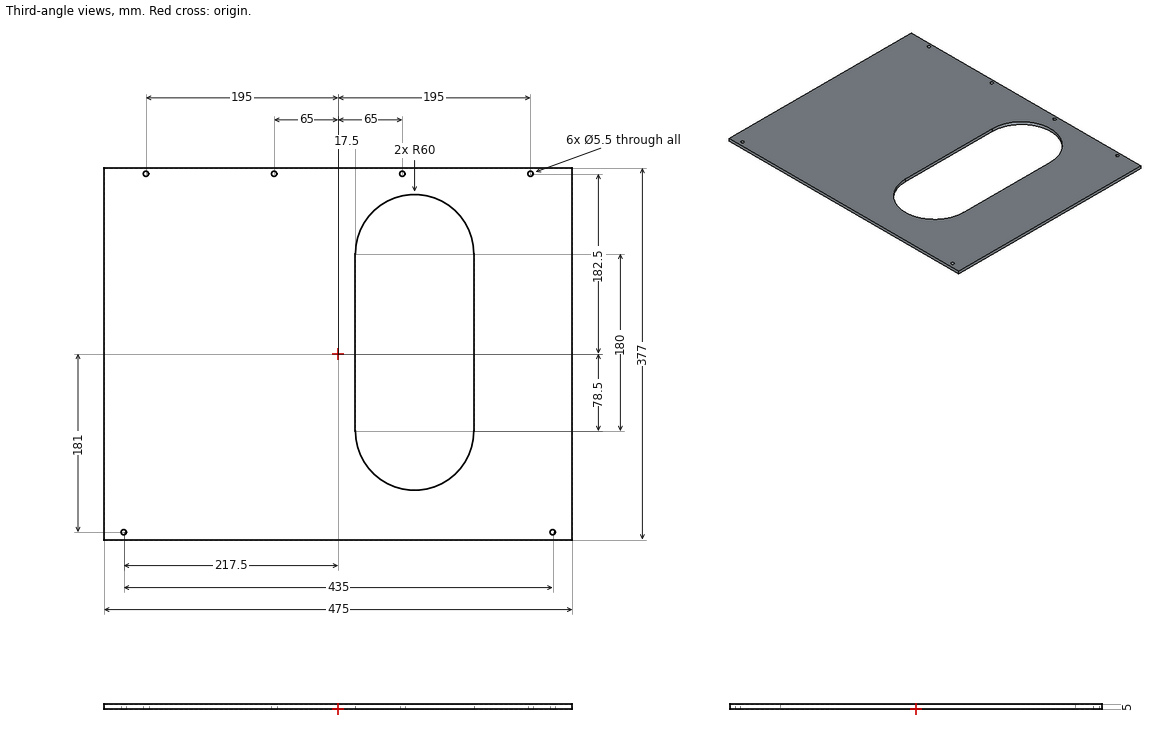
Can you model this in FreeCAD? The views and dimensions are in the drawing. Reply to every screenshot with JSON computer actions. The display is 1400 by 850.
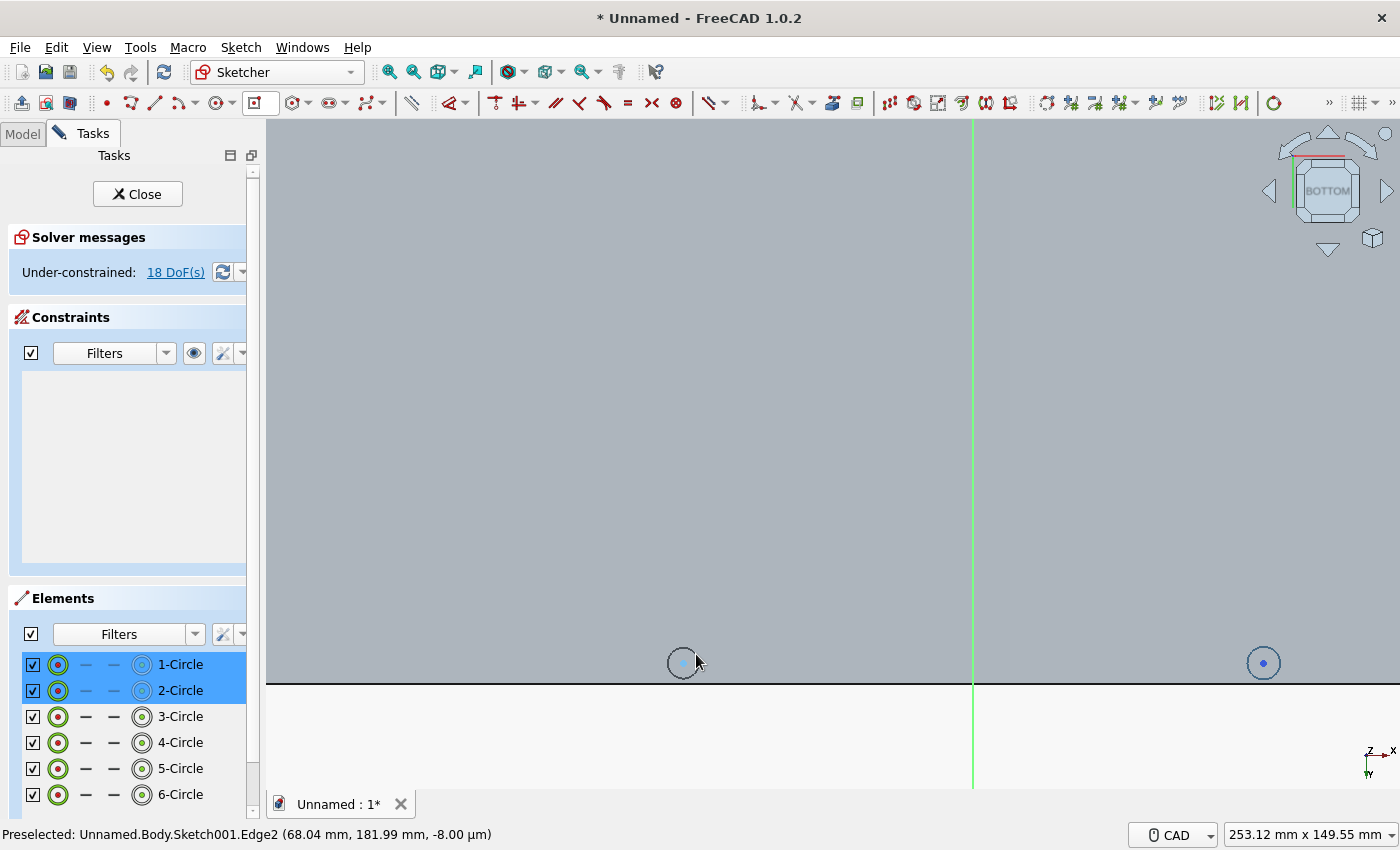
{"action": "left_click", "coordinate": [694, 652]}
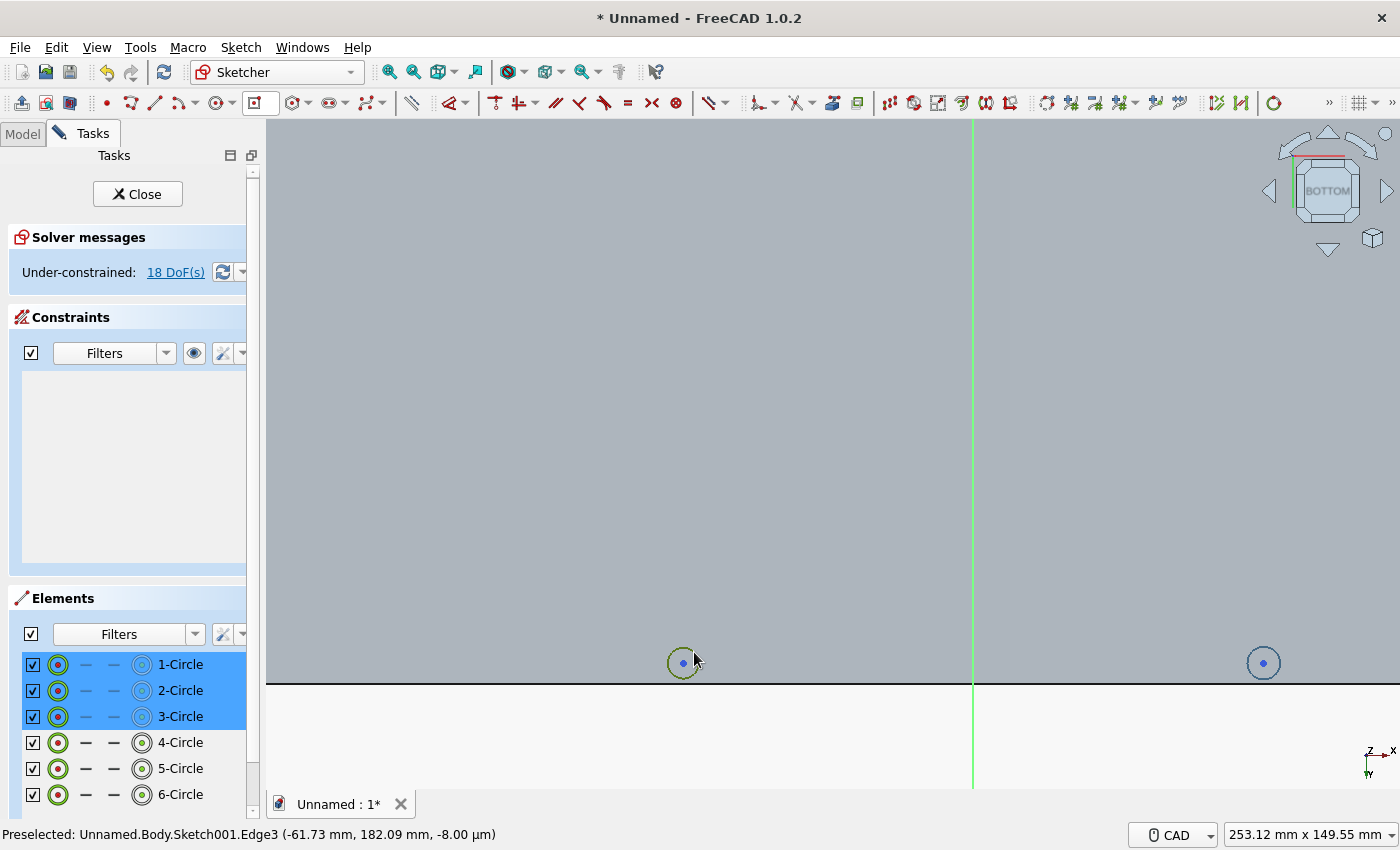
{"action": "scroll", "coordinate": [696, 654], "scroll_direction": "down", "scroll_amount": 7}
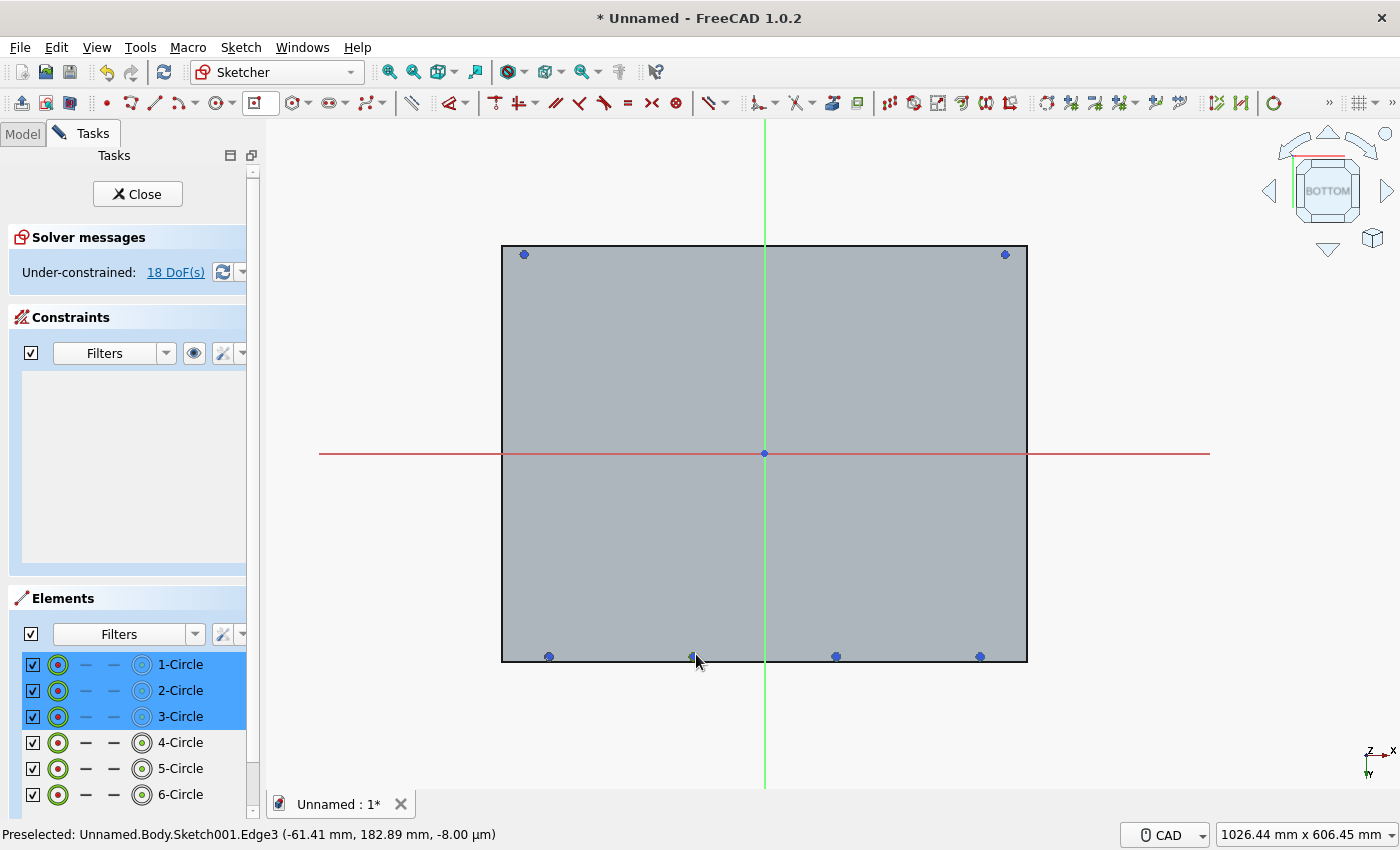
{"action": "scroll", "coordinate": [552, 654], "scroll_direction": "up", "scroll_amount": 7}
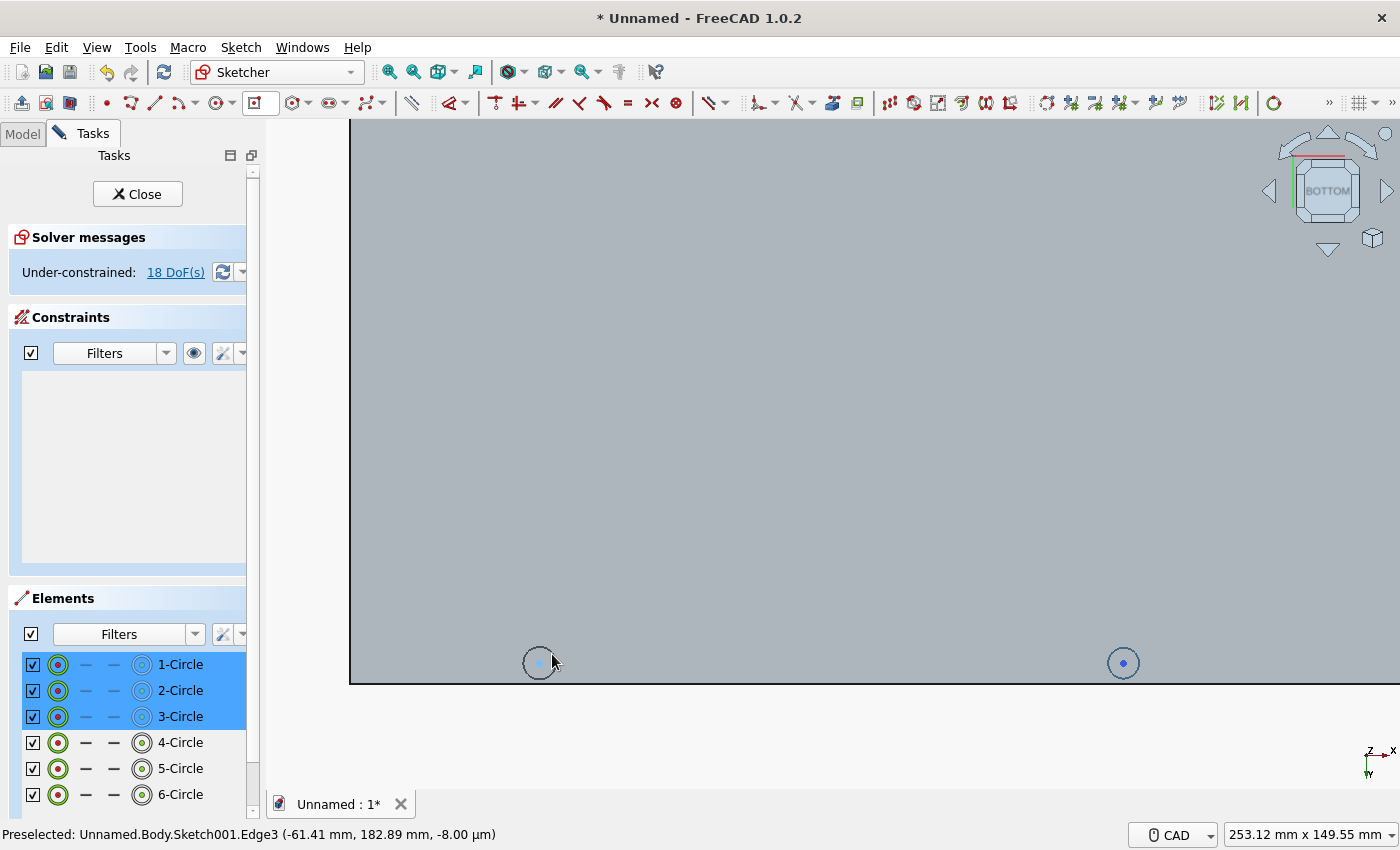
{"action": "left_click", "coordinate": [551, 652]}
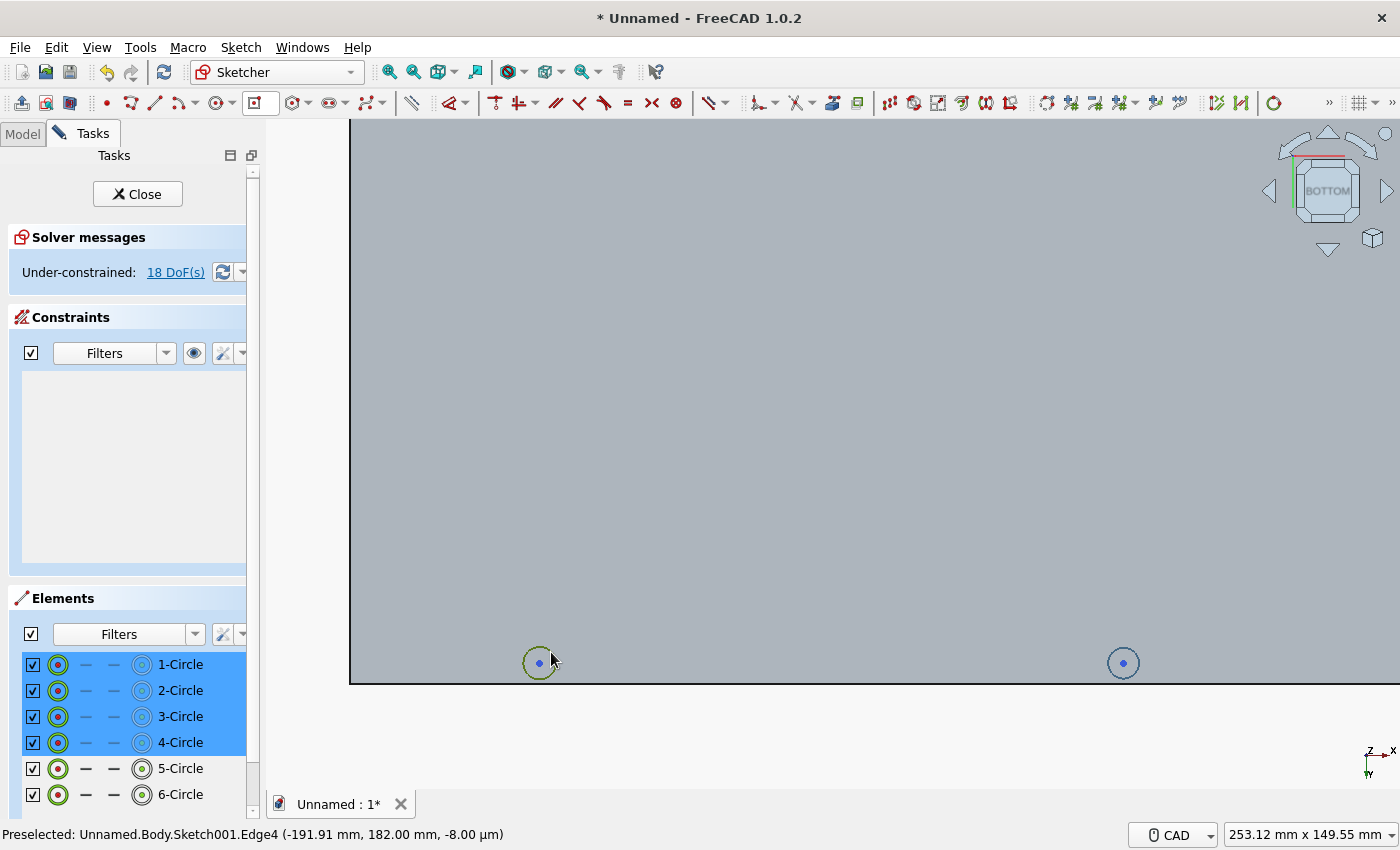
{"action": "scroll", "coordinate": [552, 654], "scroll_direction": "down", "scroll_amount": 7}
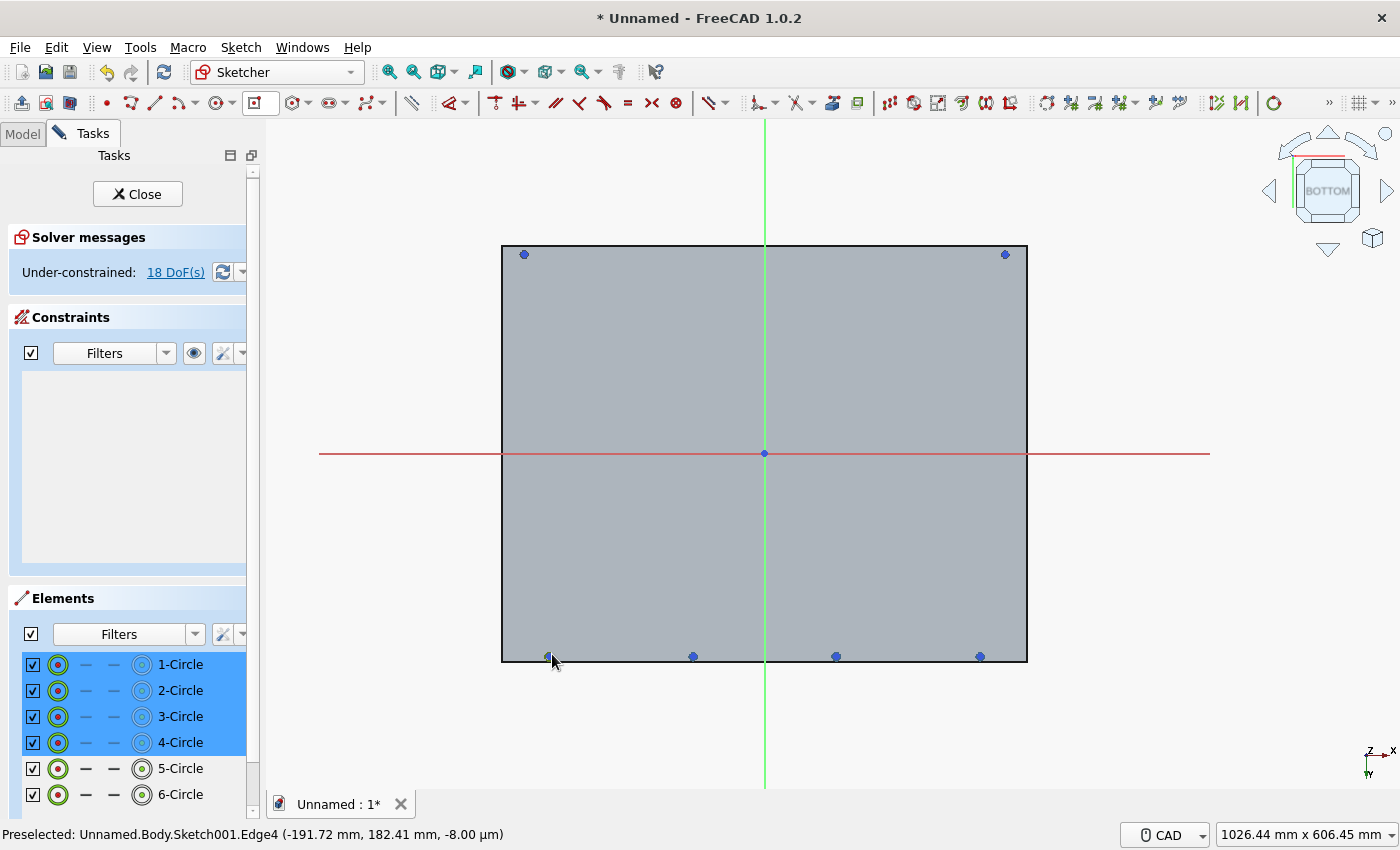
{"action": "scroll", "coordinate": [527, 252], "scroll_direction": "up", "scroll_amount": 7}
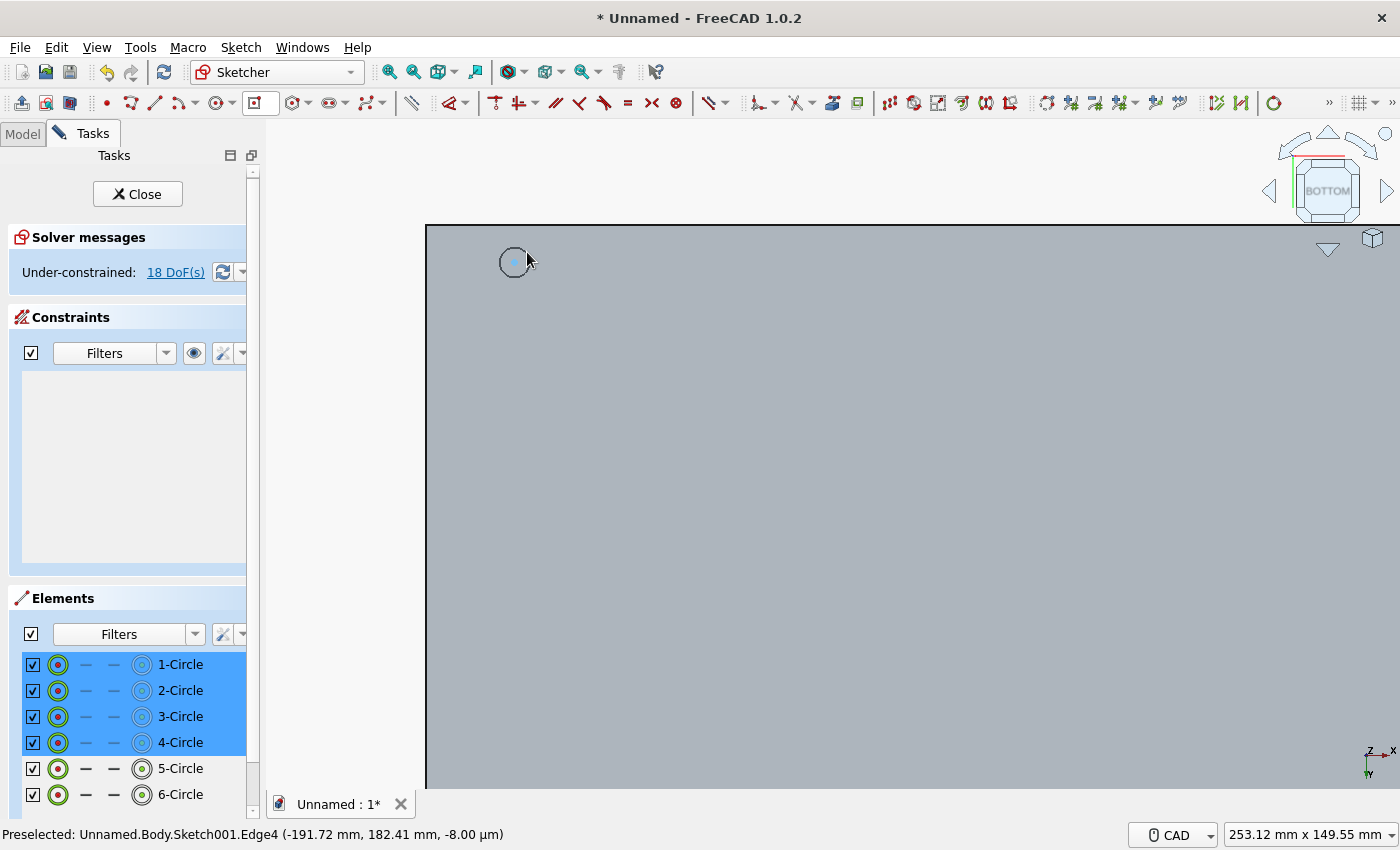
{"action": "left_click", "coordinate": [525, 252]}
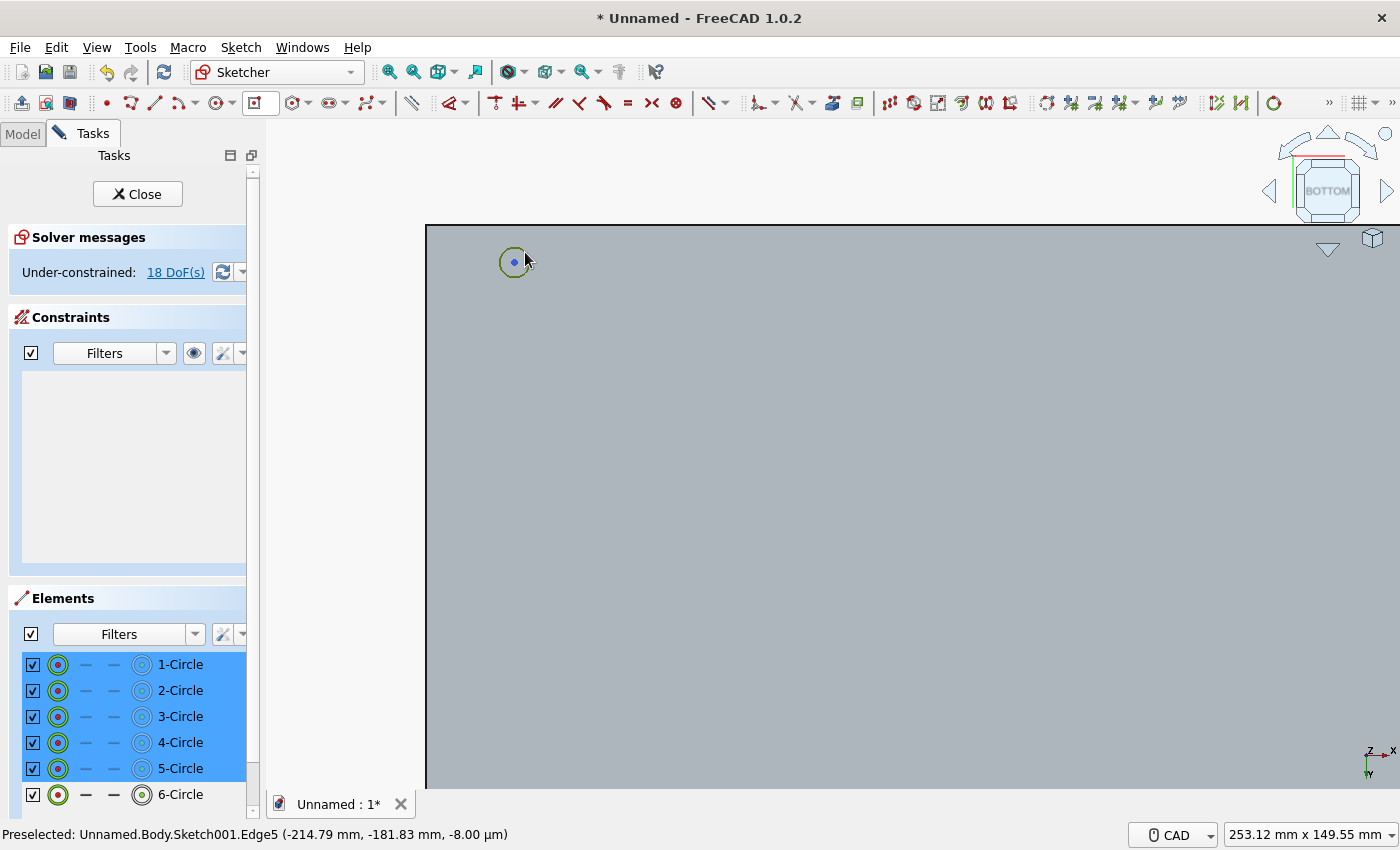
{"action": "scroll", "coordinate": [527, 251], "scroll_direction": "down", "scroll_amount": 7}